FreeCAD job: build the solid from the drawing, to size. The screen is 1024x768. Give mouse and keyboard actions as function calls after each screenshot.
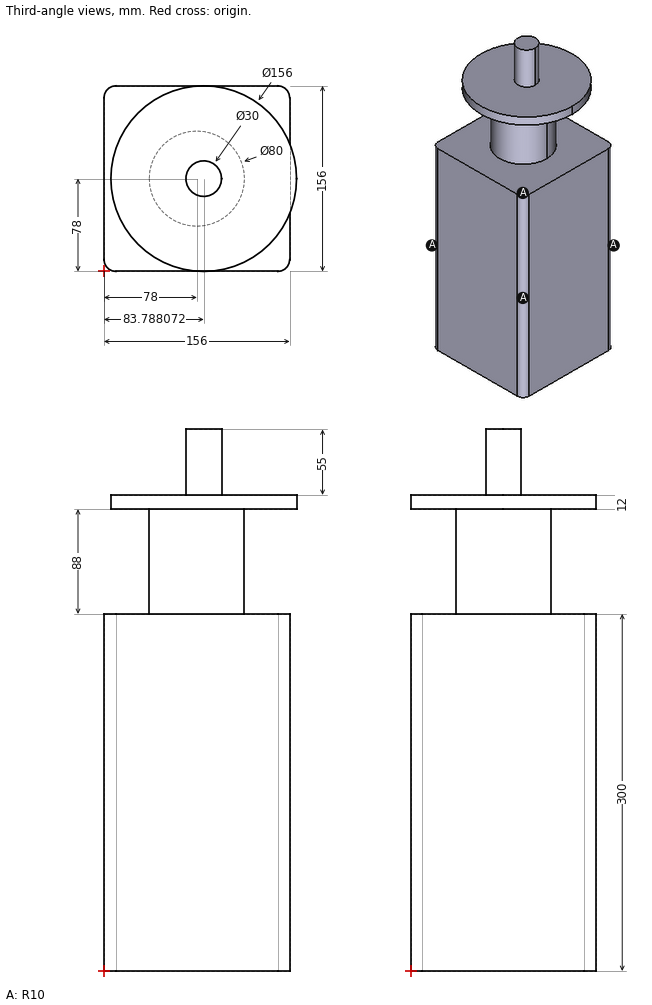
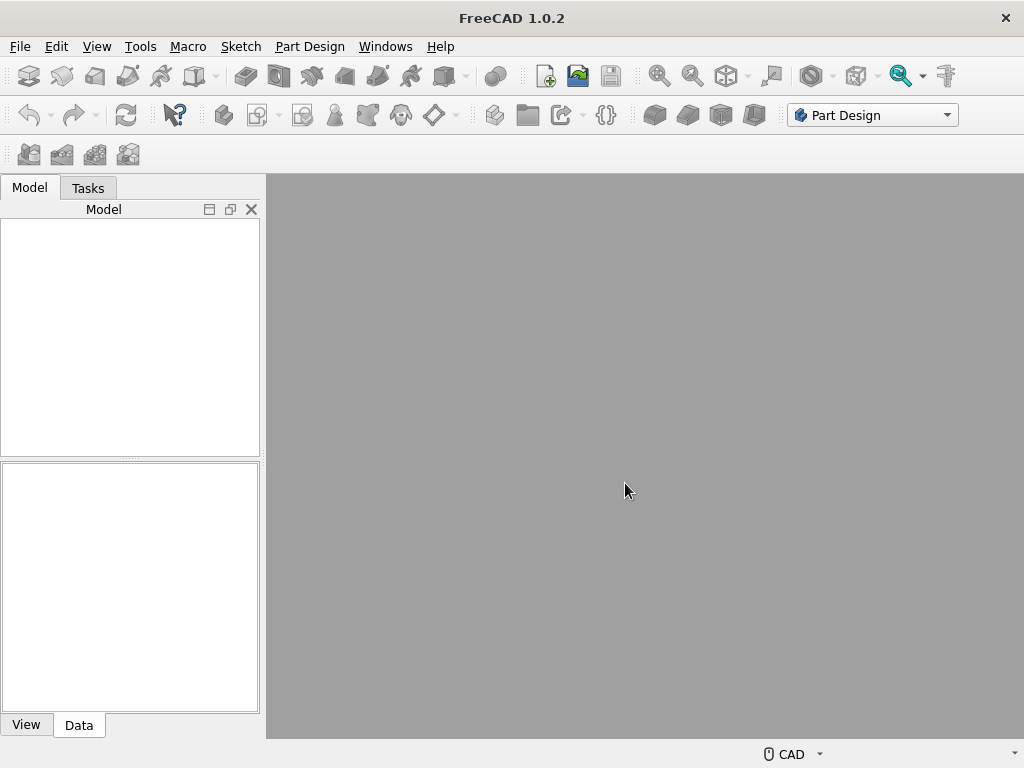
click(545, 76)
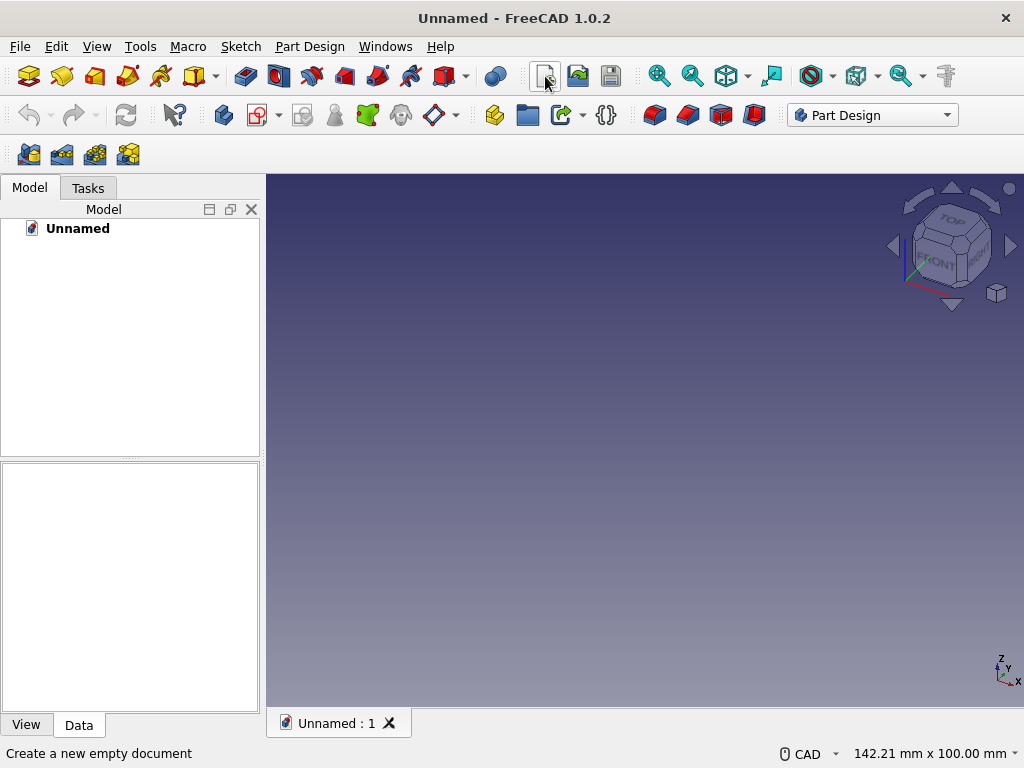
click(256, 116)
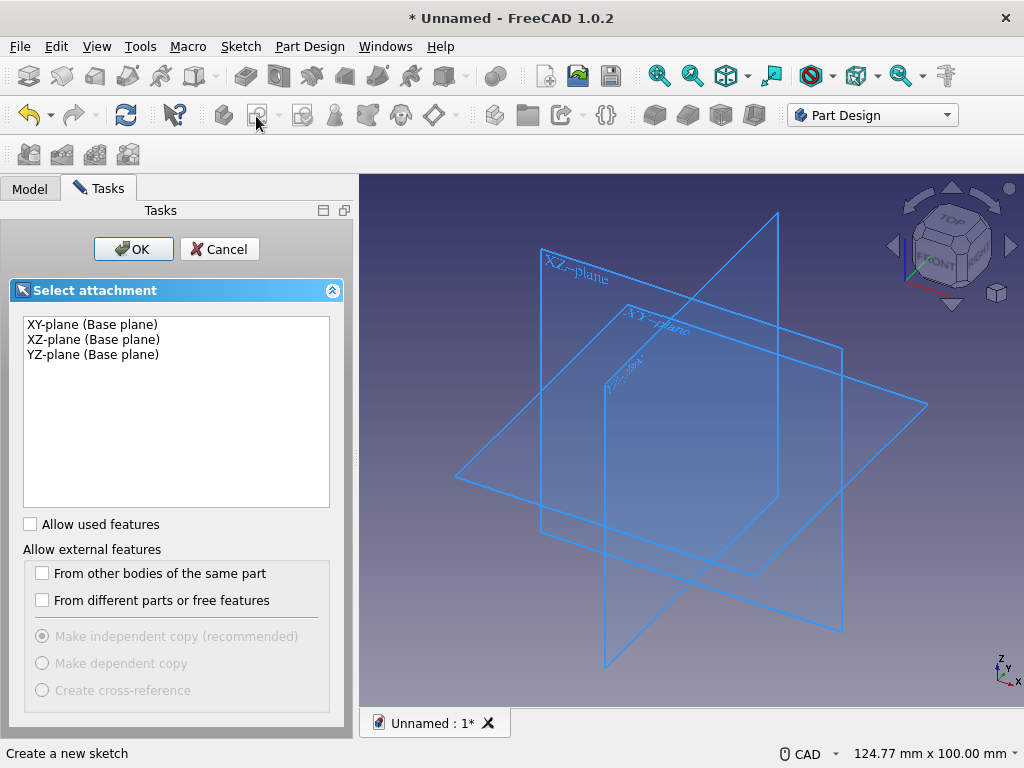
click(84, 324)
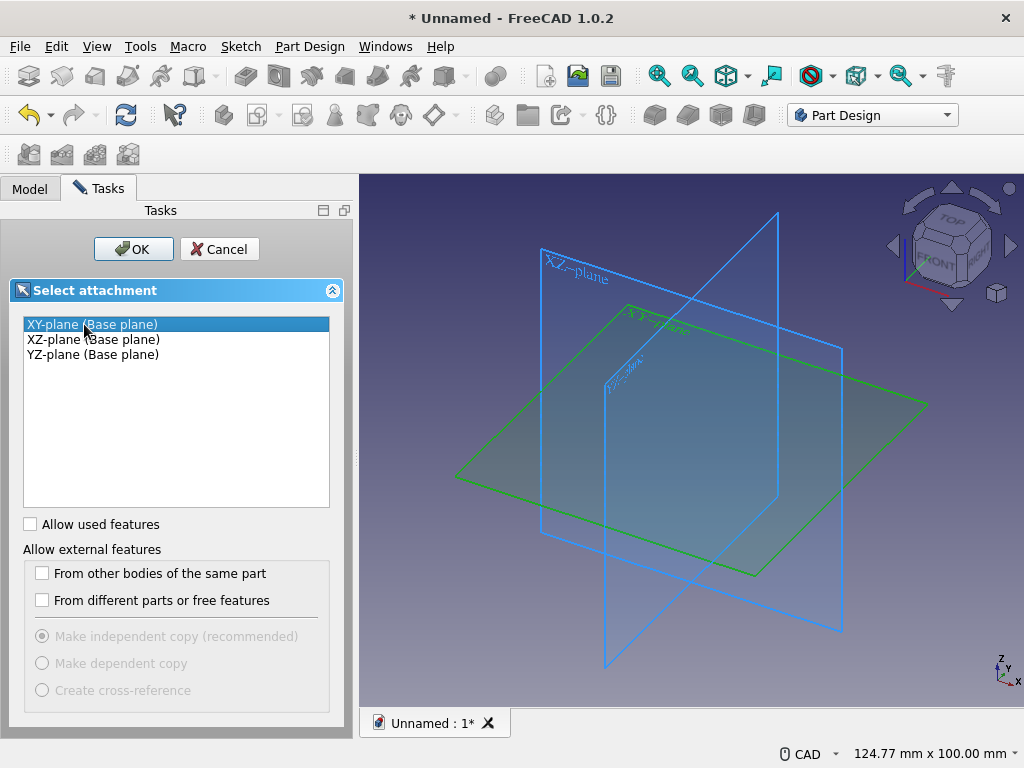
click(134, 249)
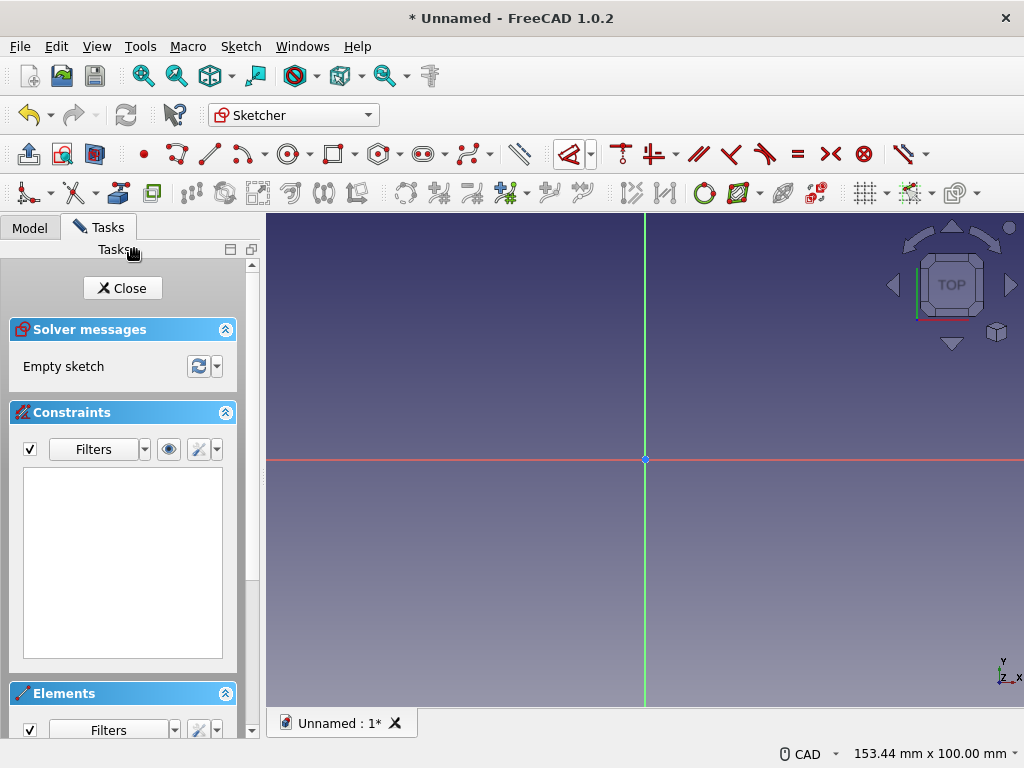
scroll(312, 679, down, 5)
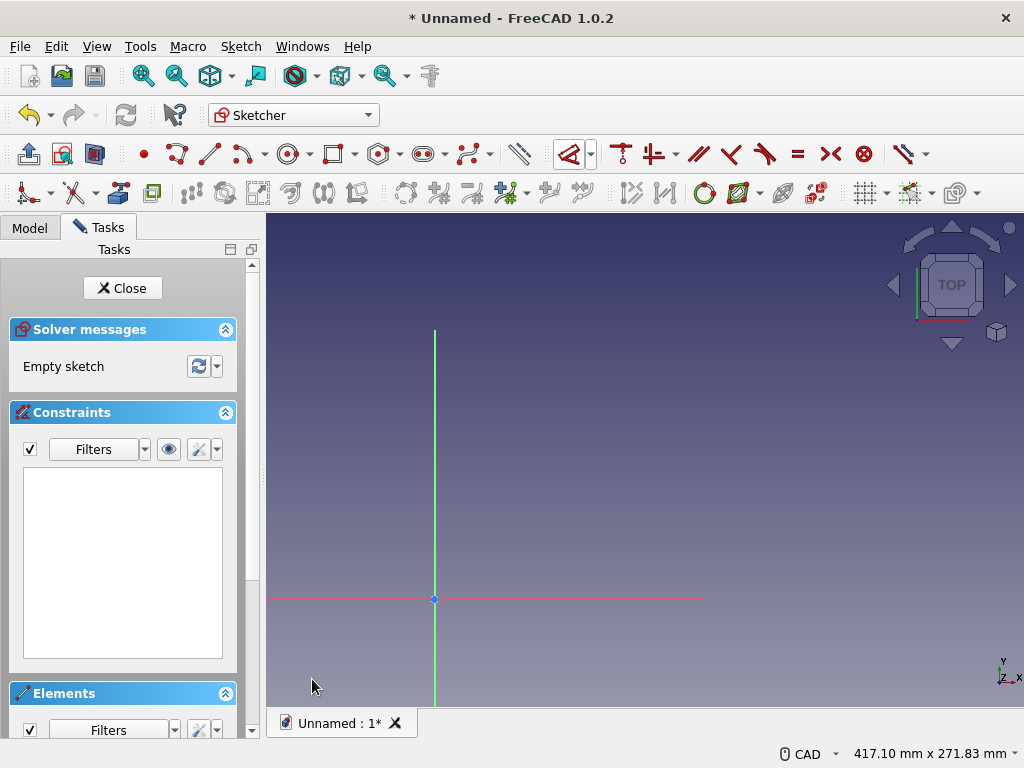
click(332, 154)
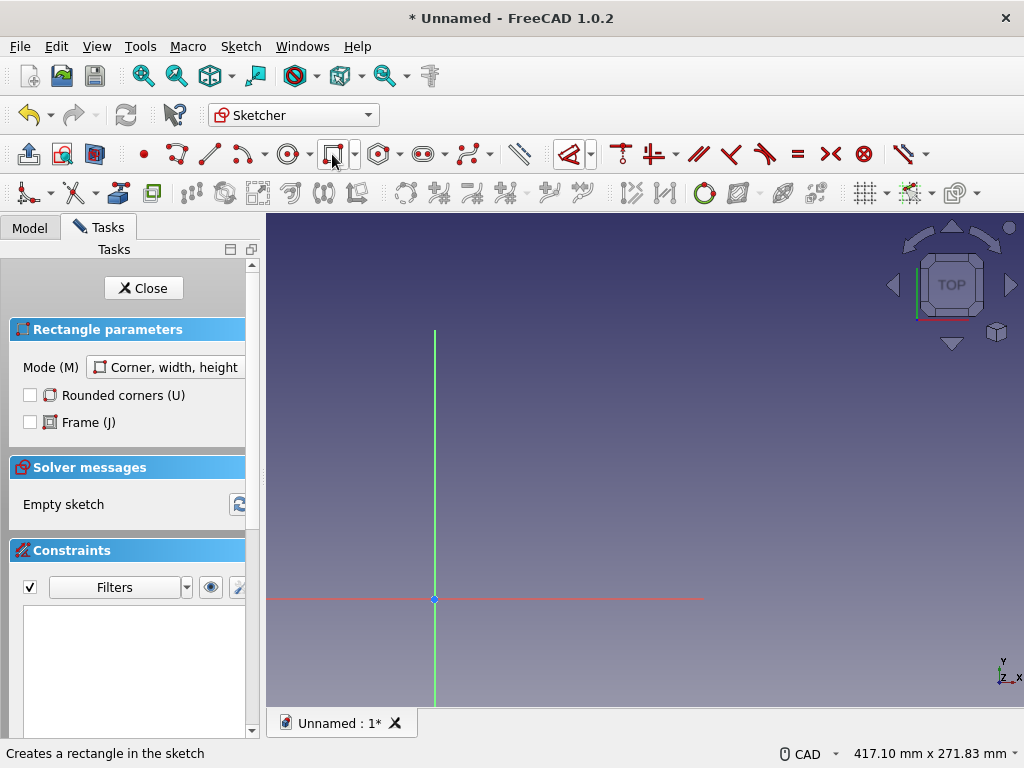
click(435, 599)
move(718, 316)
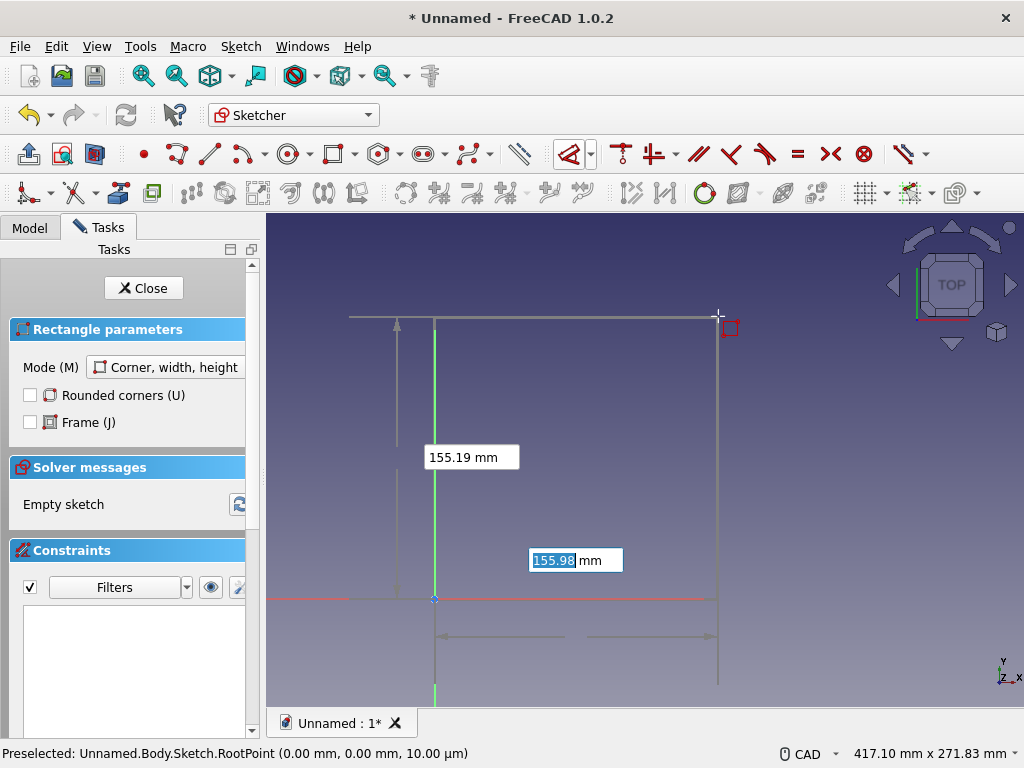
text(156)
key(Tab)
text(156)
key(Return)
key(Escape)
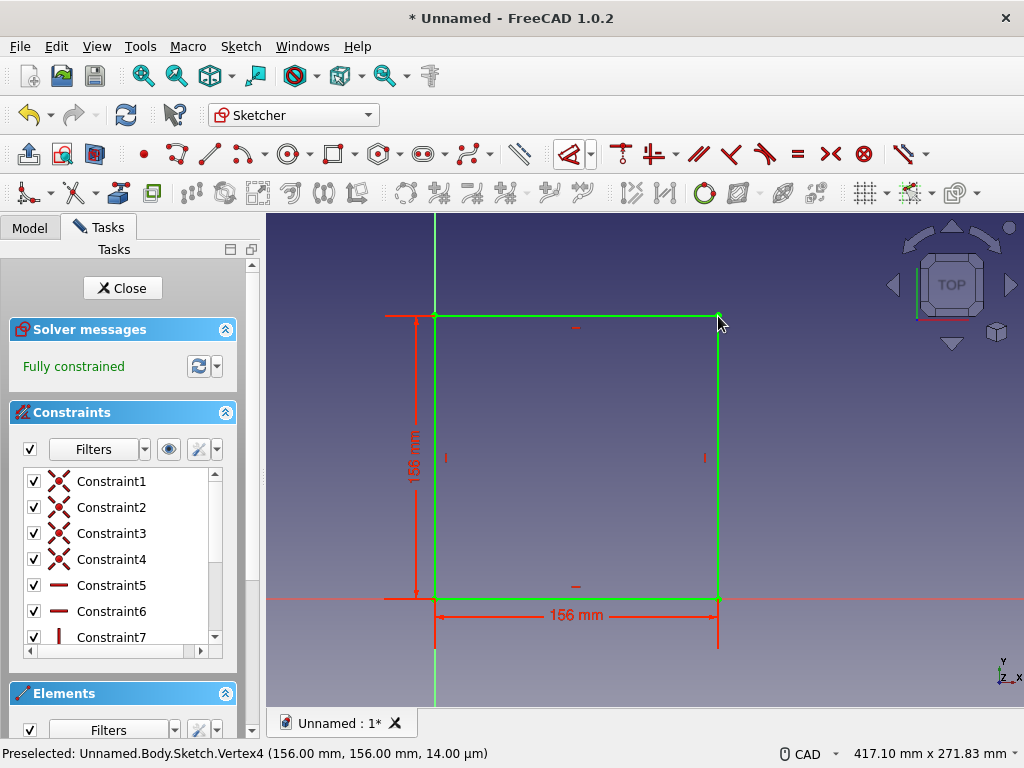
click(123, 288)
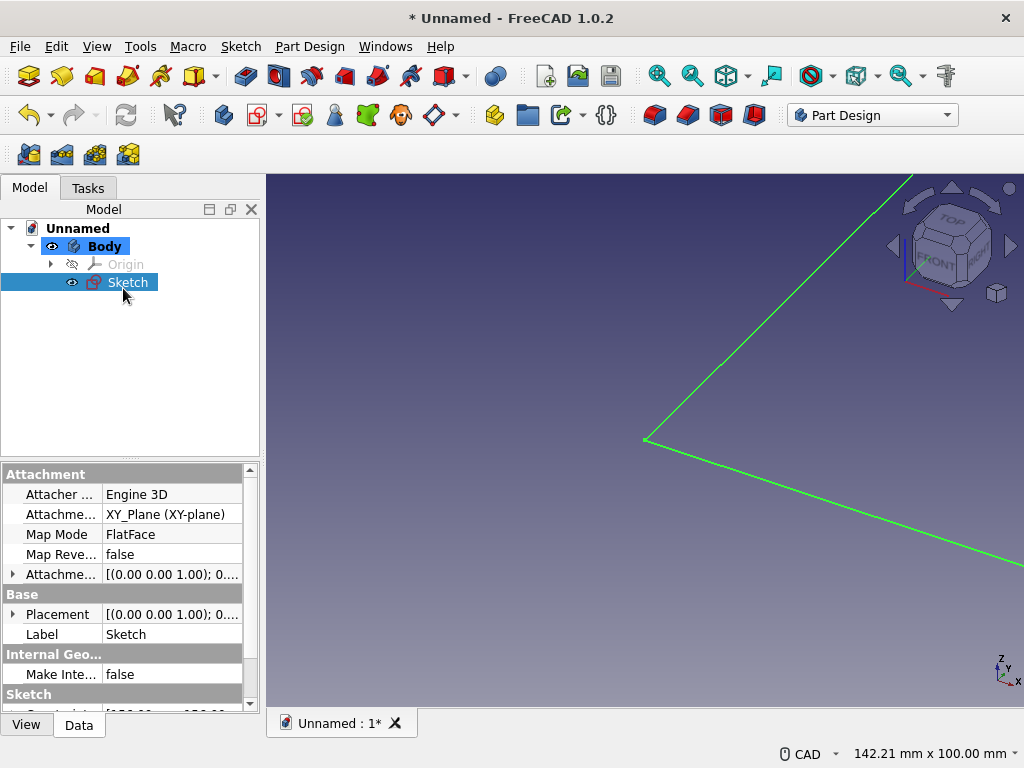
click(29, 76)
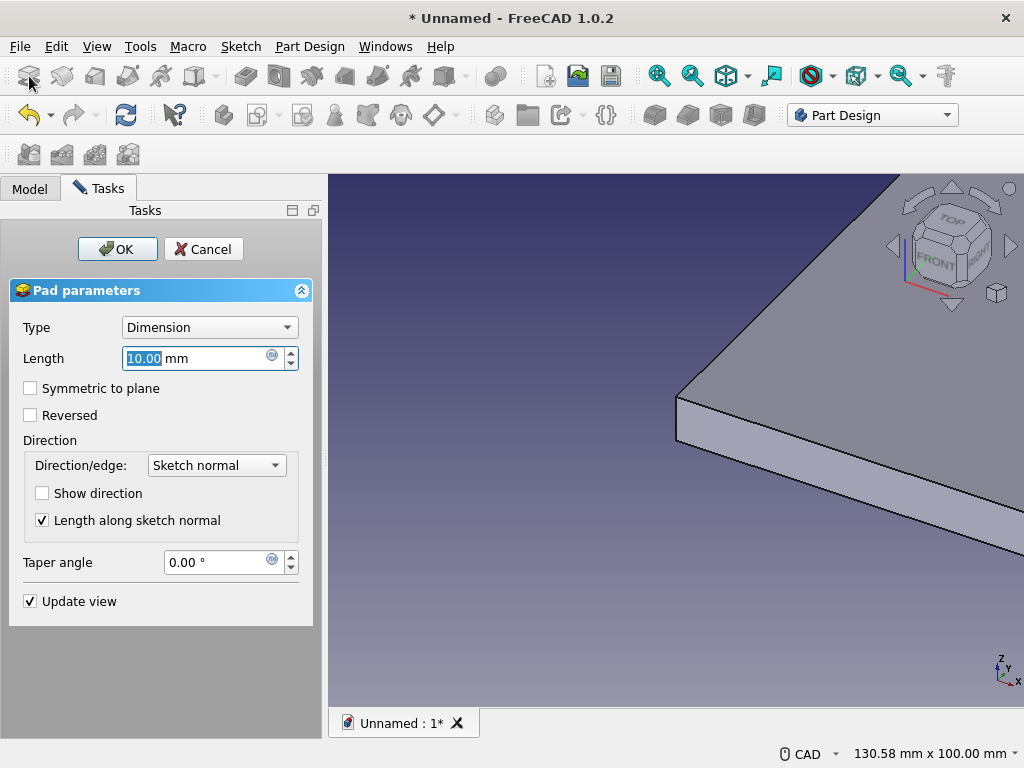
text(300)
key(Tab)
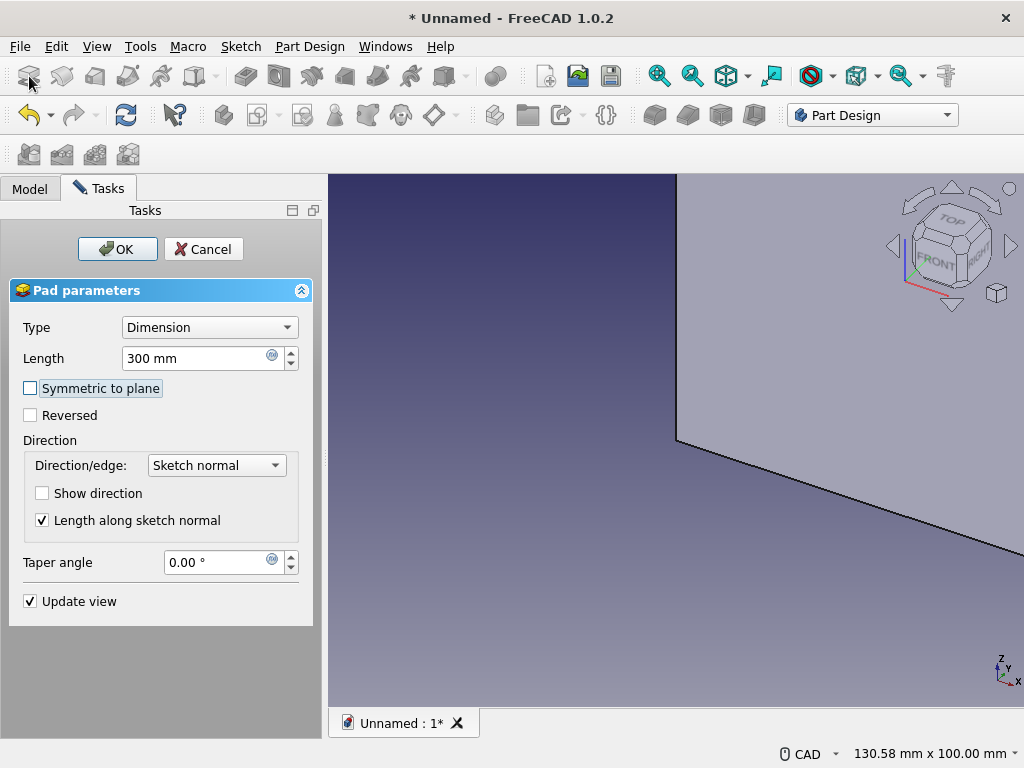
click(118, 249)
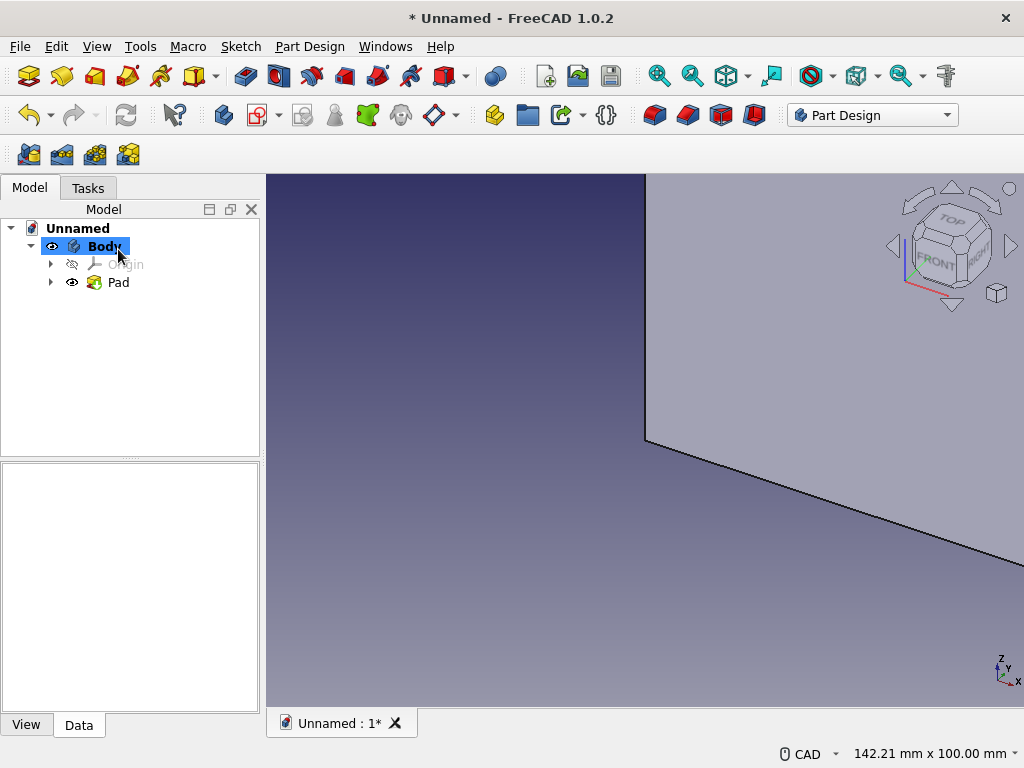
click(660, 76)